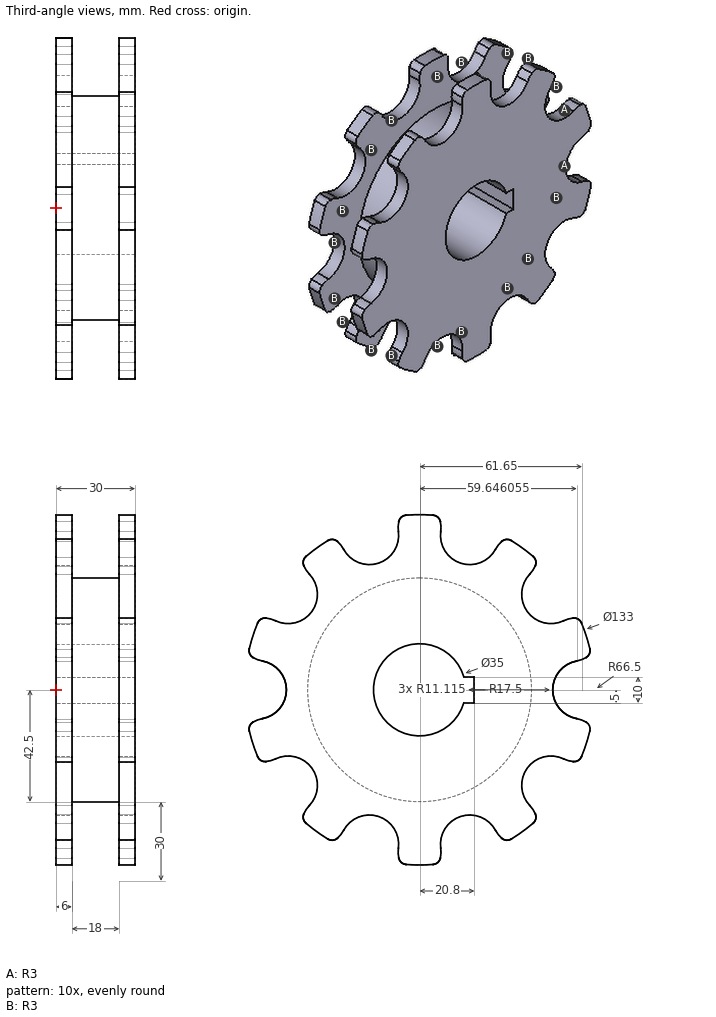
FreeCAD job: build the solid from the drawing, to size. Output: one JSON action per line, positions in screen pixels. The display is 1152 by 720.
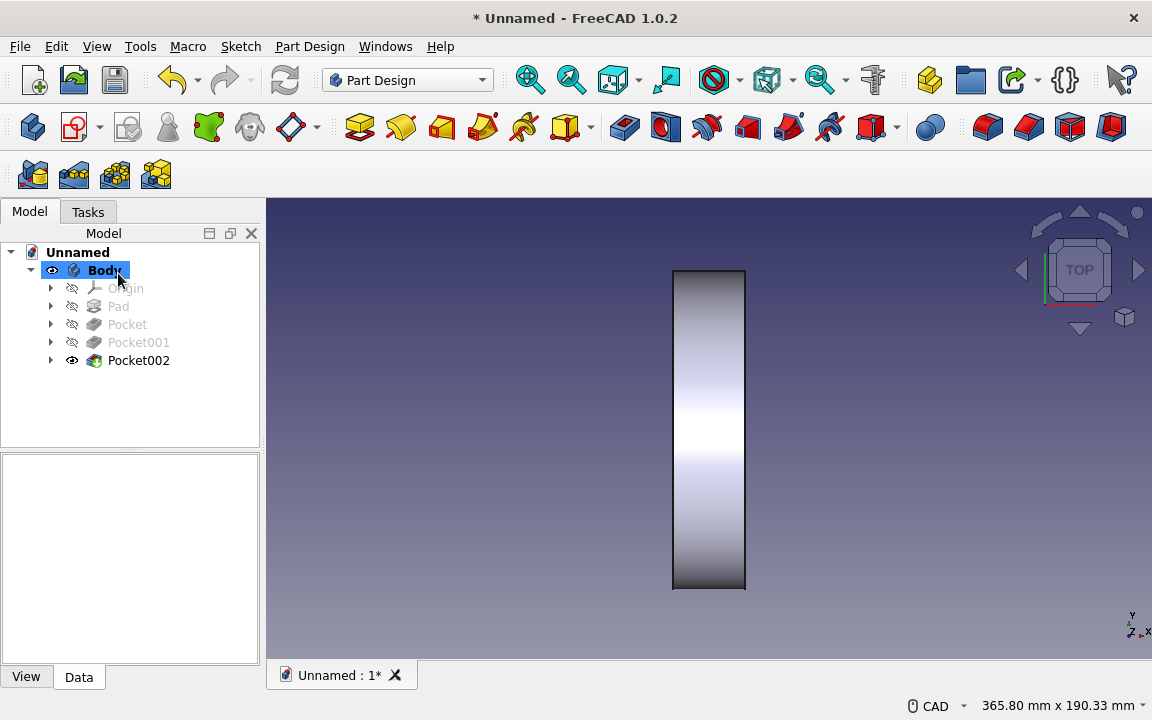
{"action": "key", "text": "1"}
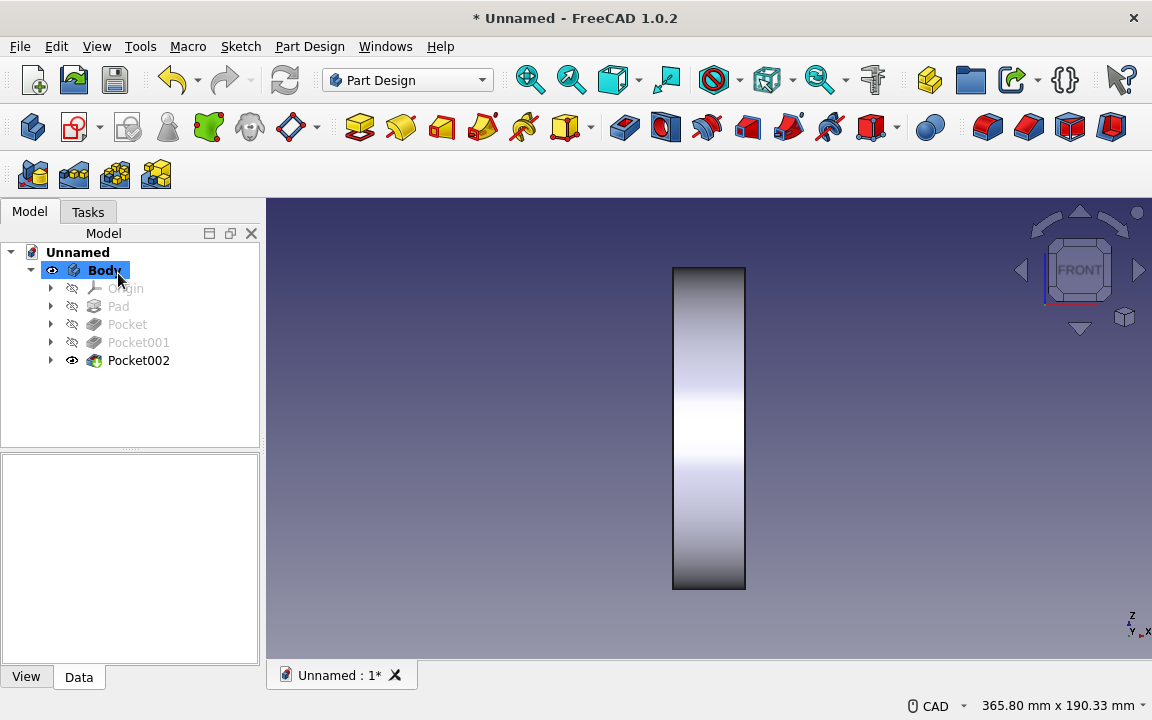
{"action": "key", "text": "3"}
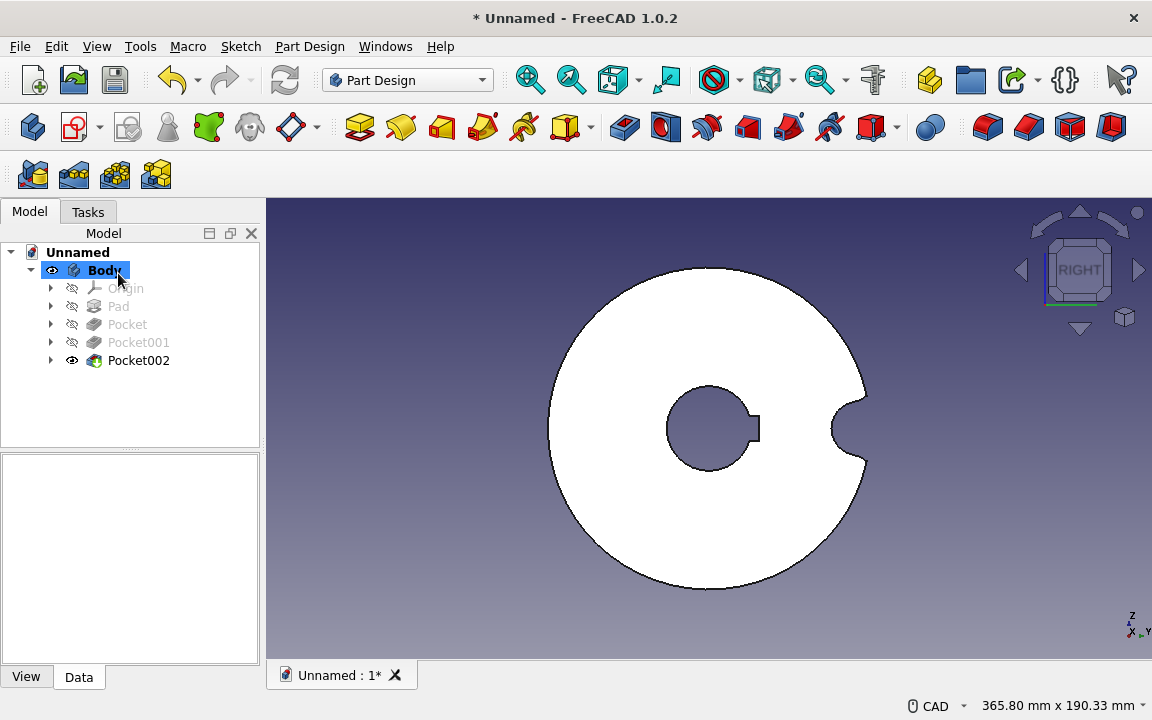
{"action": "key", "text": "5"}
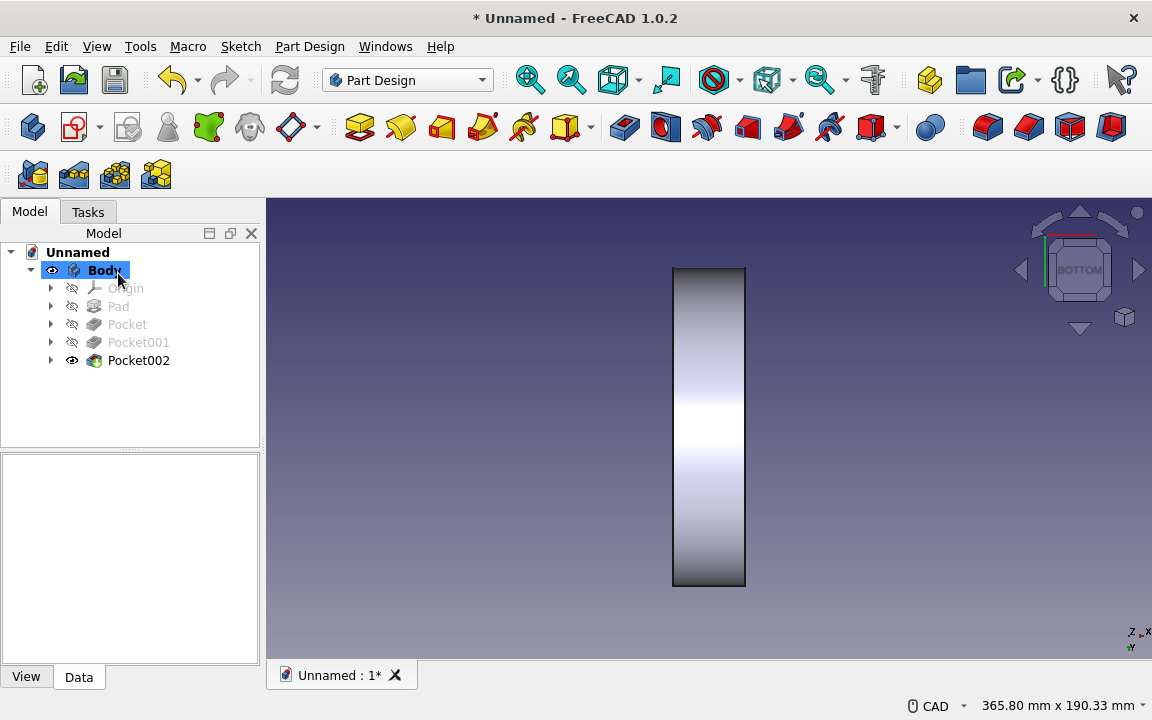
{"action": "key", "text": "4"}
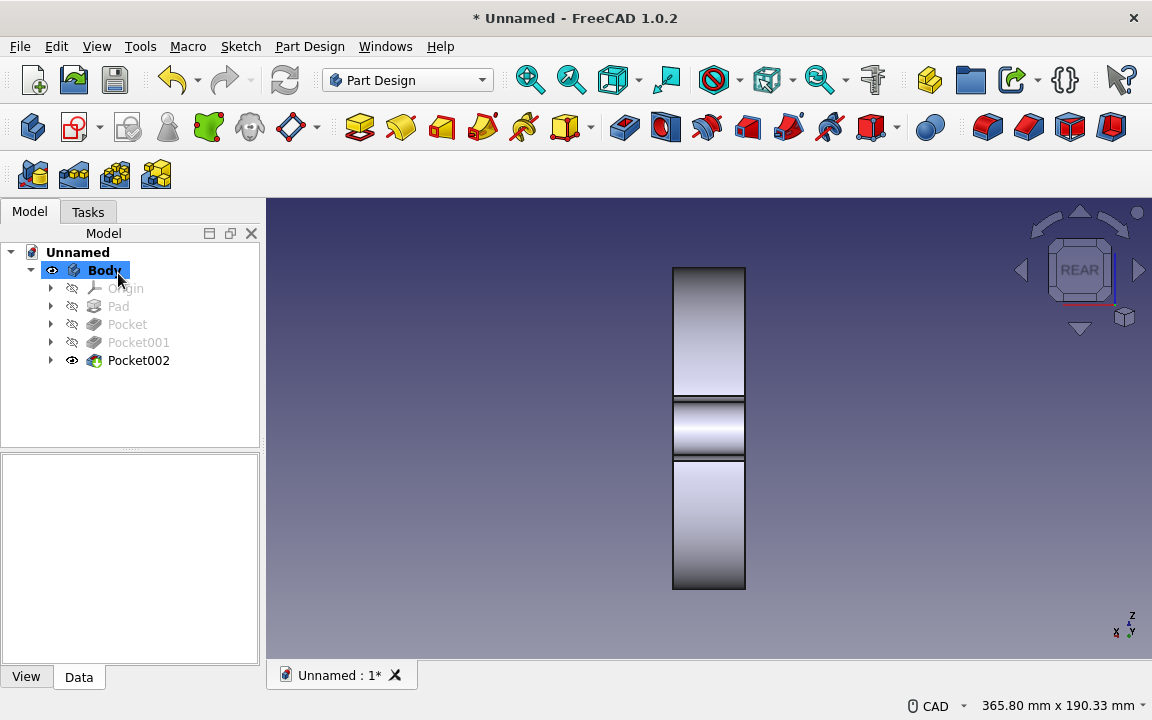
{"action": "left_click", "coordinate": [709, 395]}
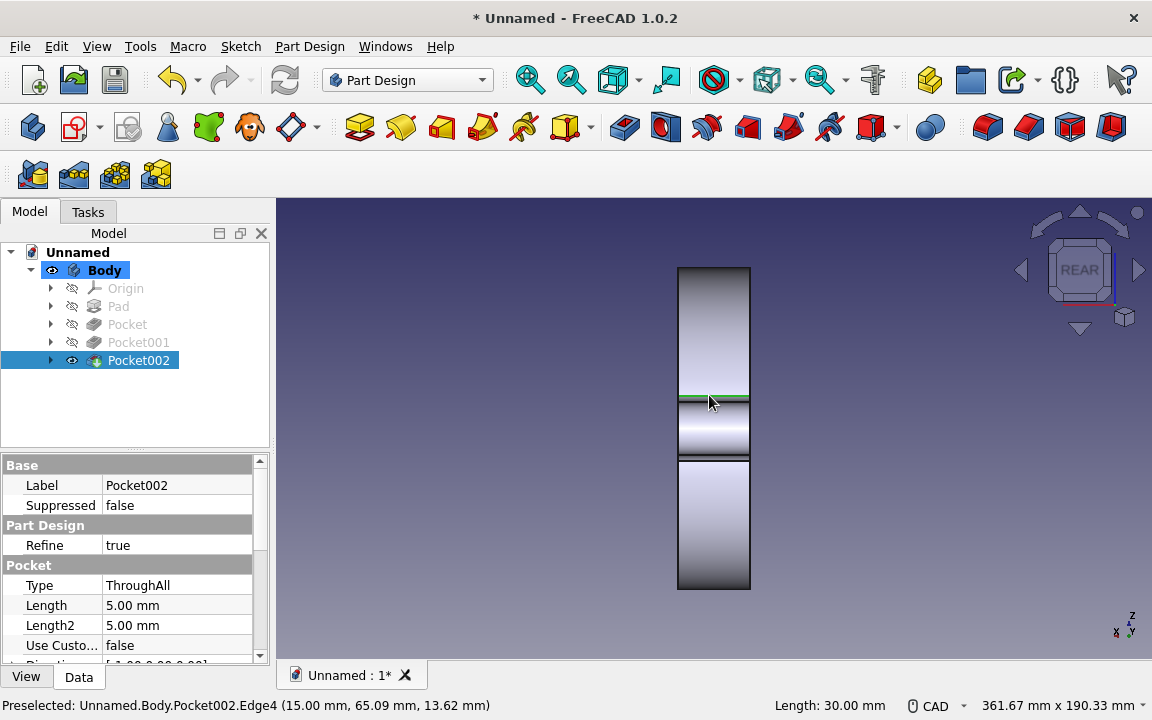
{"action": "left_click", "coordinate": [714, 460], "text": "ctrl"}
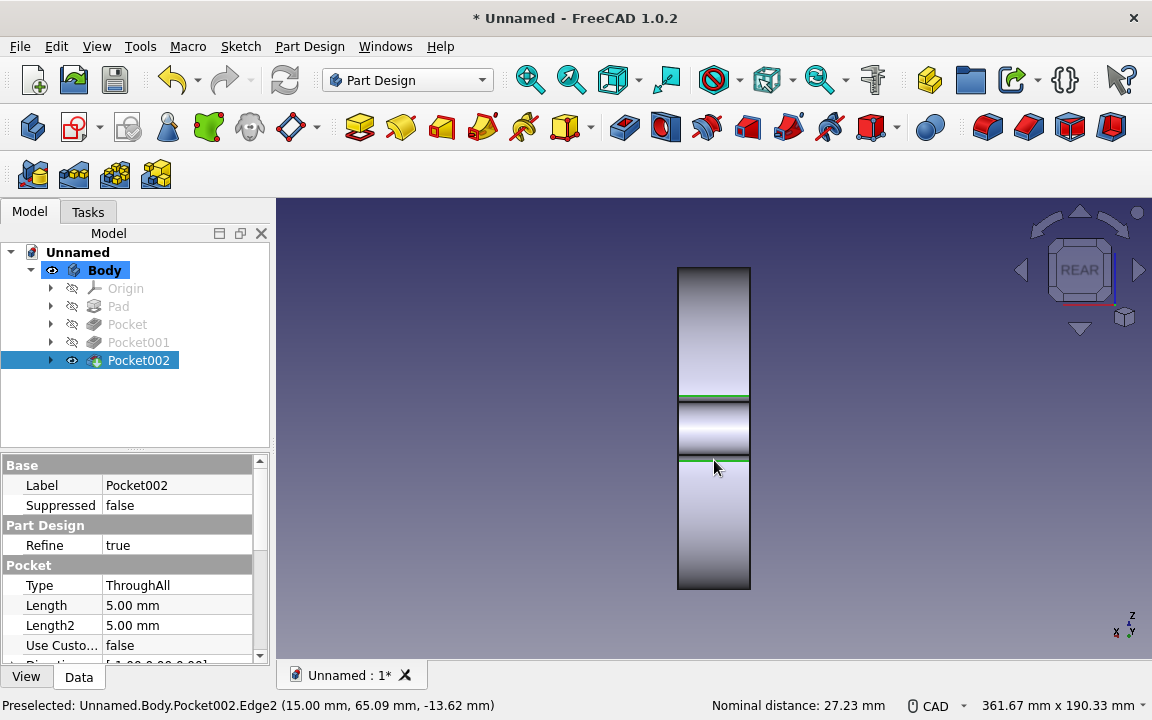
{"action": "left_click", "coordinate": [988, 128]}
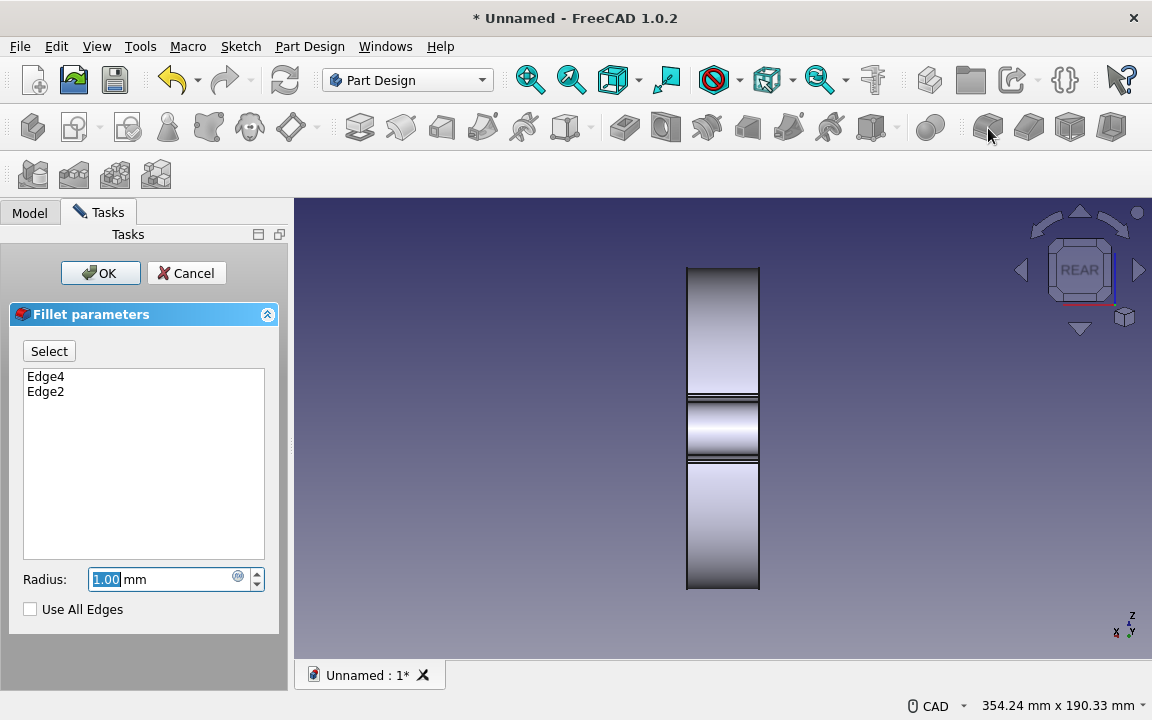
{"action": "type", "text": "3"}
{"action": "key", "text": "Tab"}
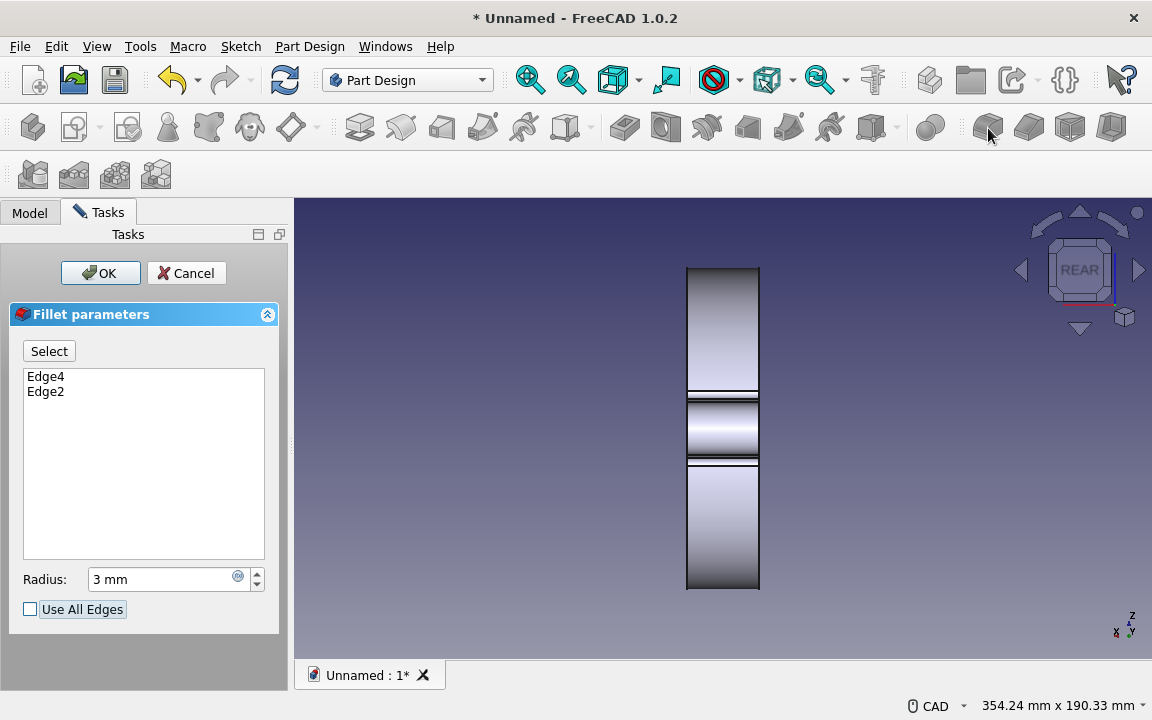
{"action": "left_click", "coordinate": [101, 273]}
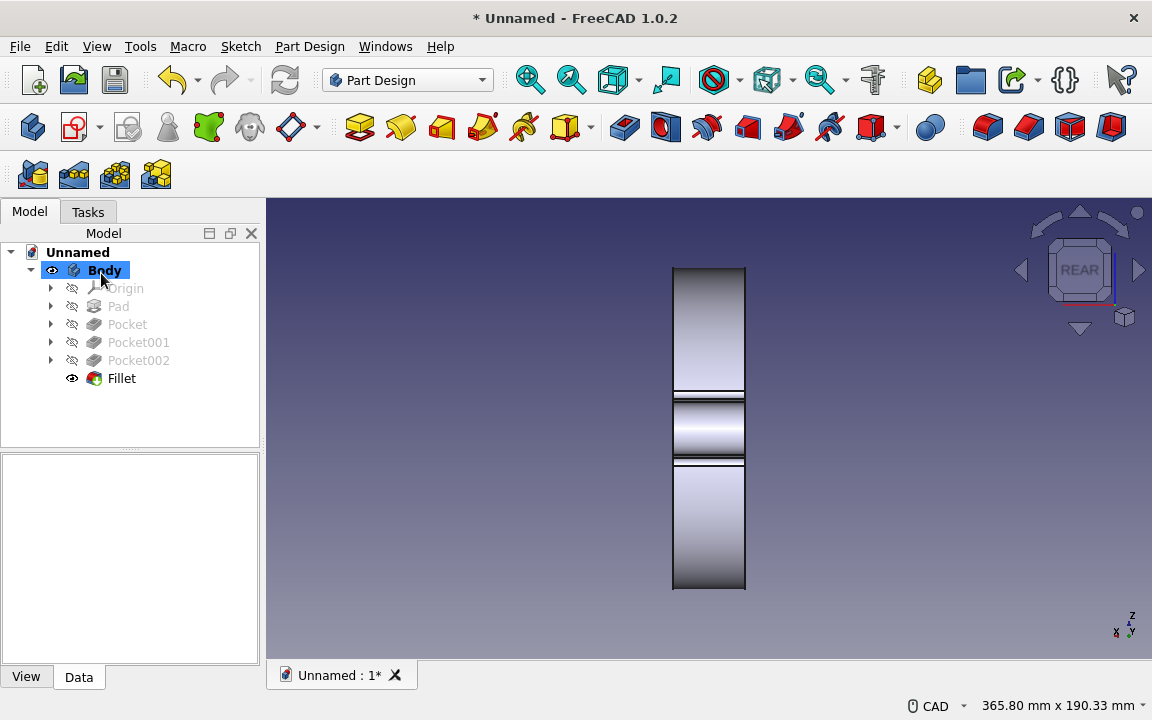
{"action": "left_click", "coordinate": [117, 360]}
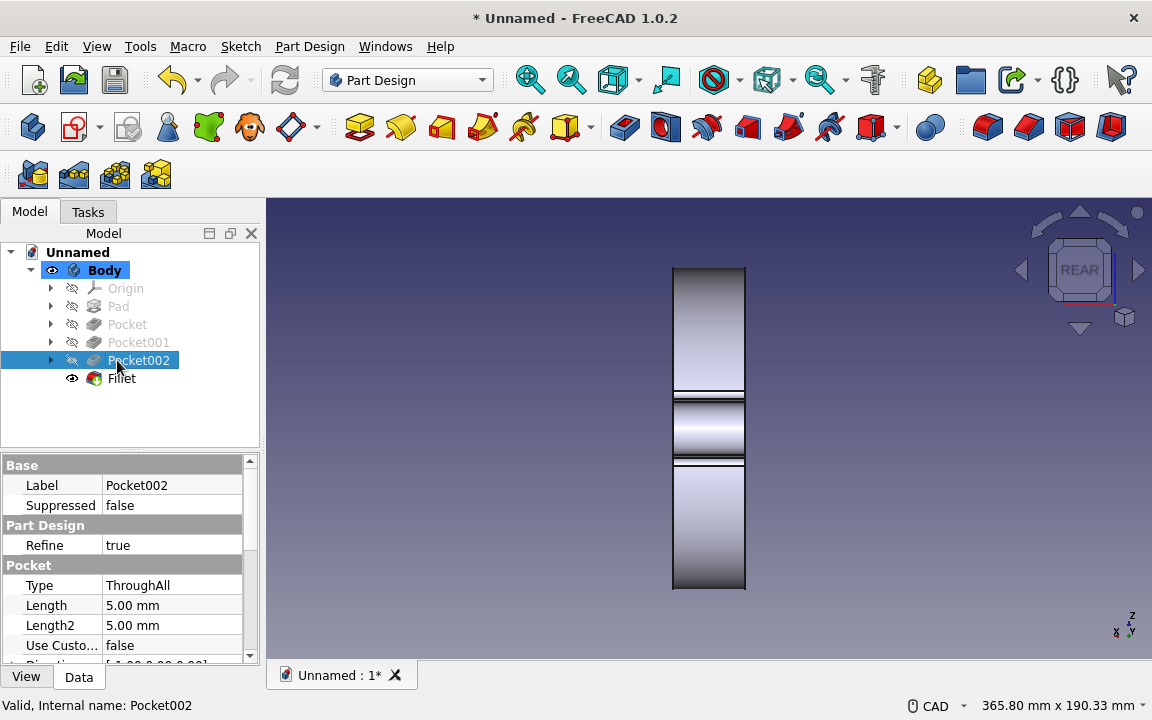
{"action": "left_click", "coordinate": [115, 174]}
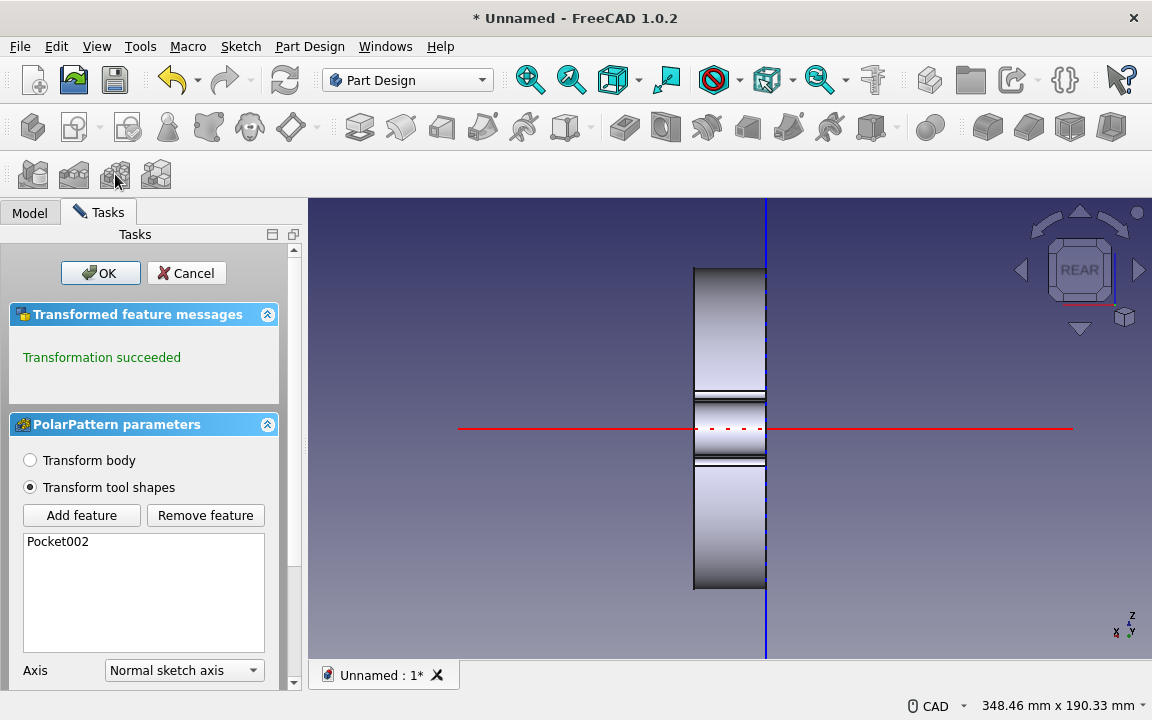
{"action": "left_click", "coordinate": [185, 670]}